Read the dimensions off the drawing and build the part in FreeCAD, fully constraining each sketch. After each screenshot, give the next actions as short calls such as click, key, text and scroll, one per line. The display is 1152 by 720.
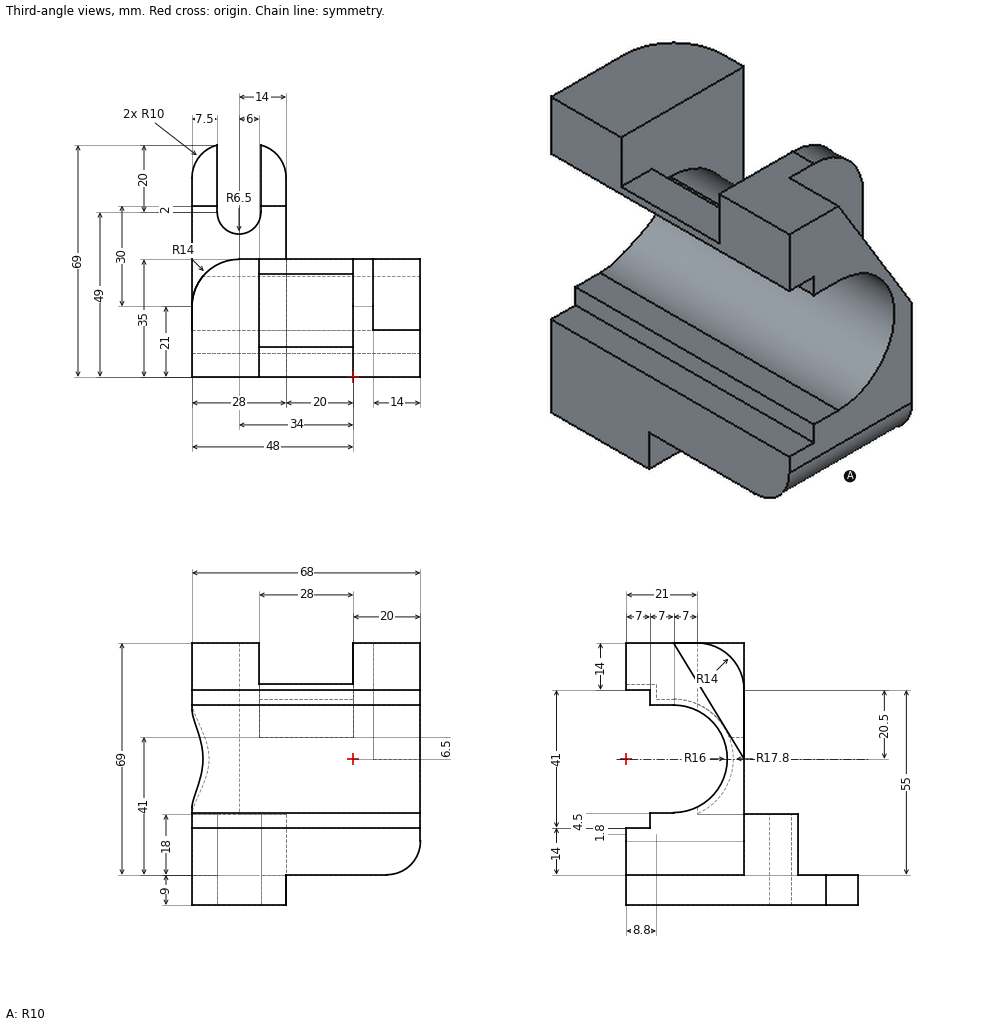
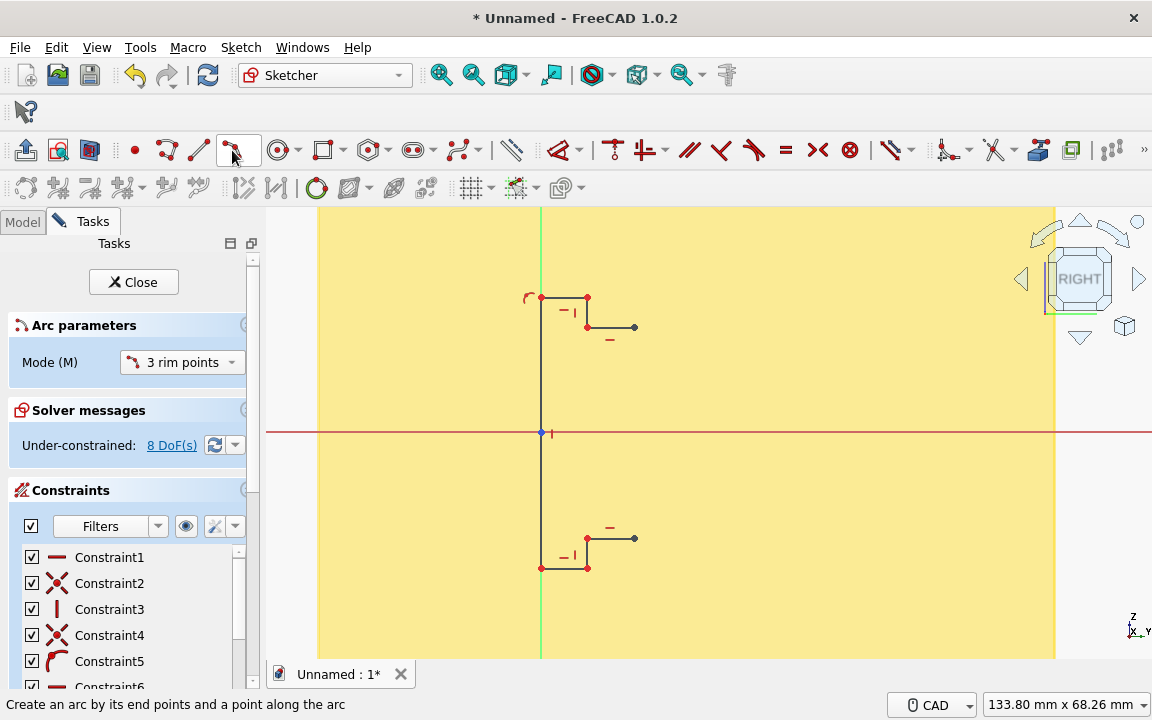
click(634, 539)
click(634, 328)
click(735, 465)
key(Escape)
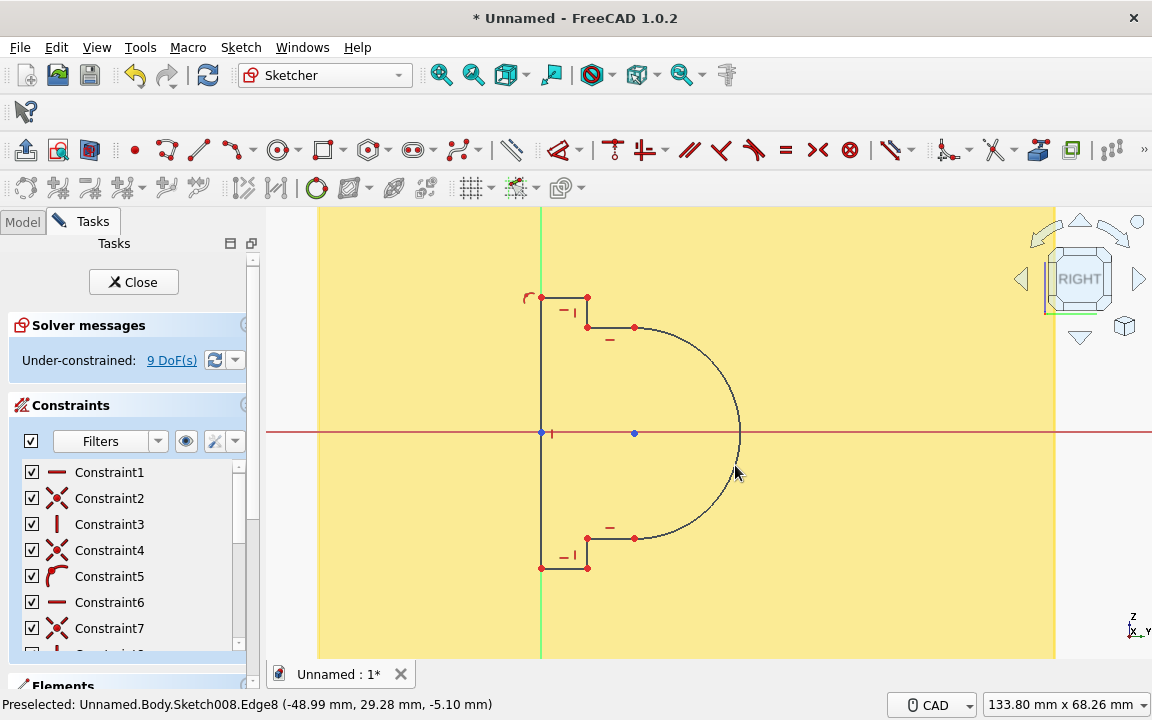
click(620, 328)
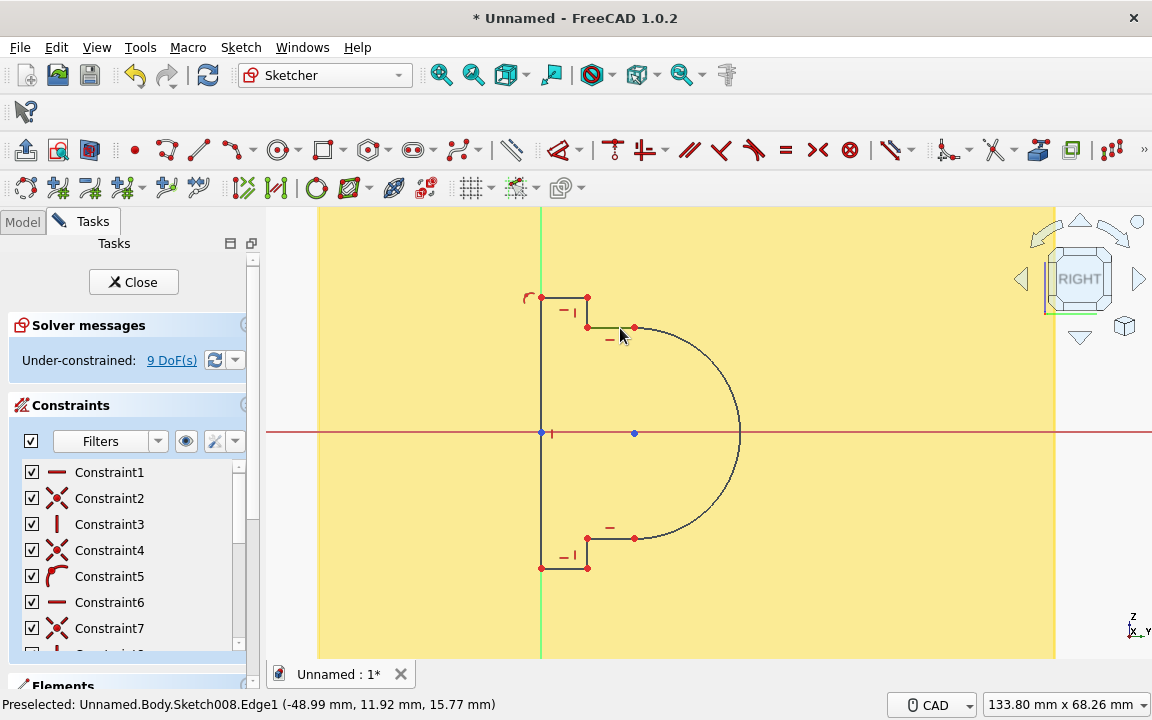
click(720, 496)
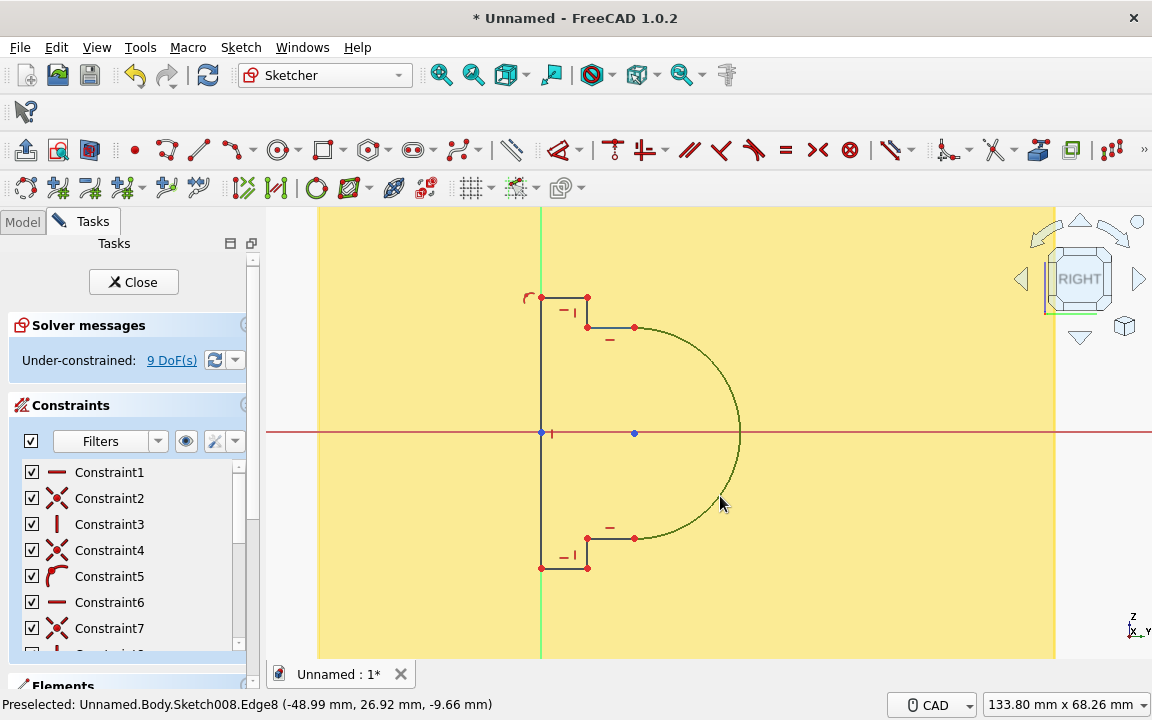
click(754, 150)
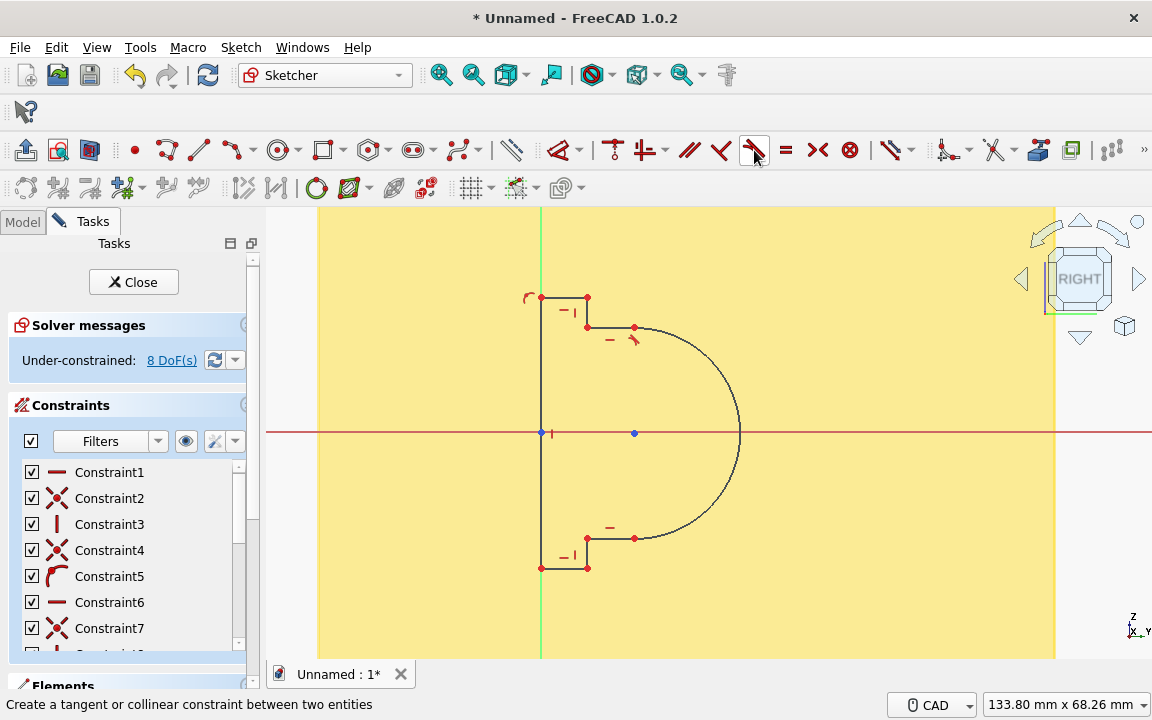
click(601, 539)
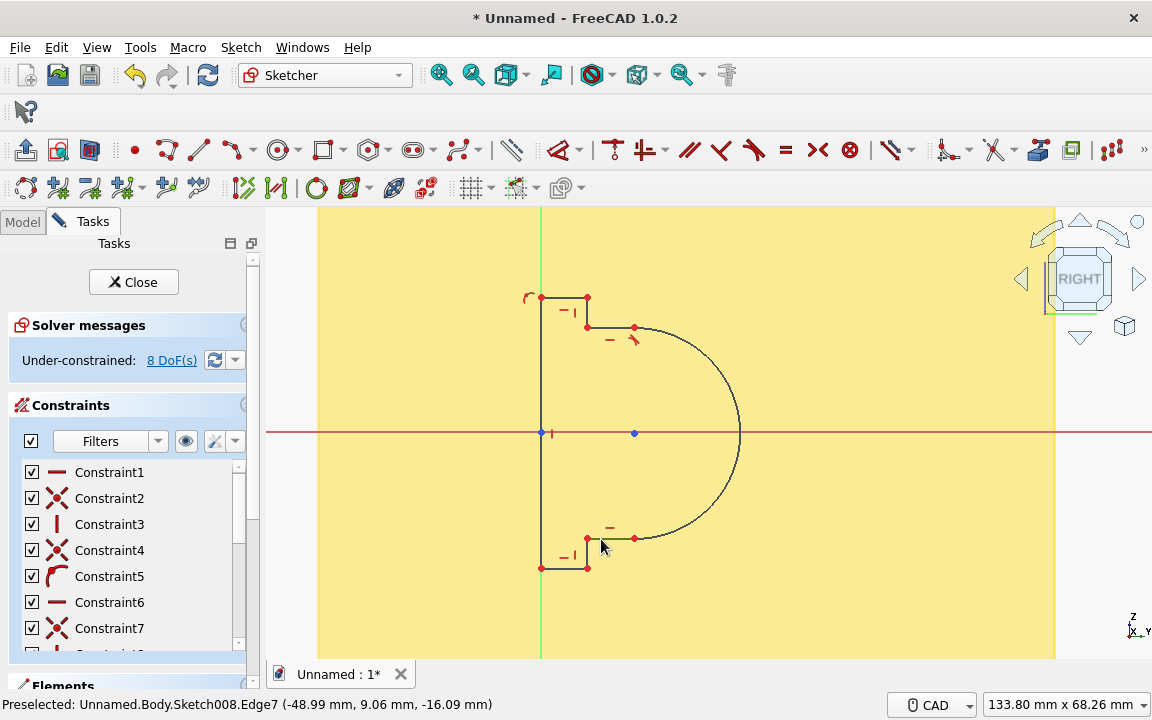
click(720, 496)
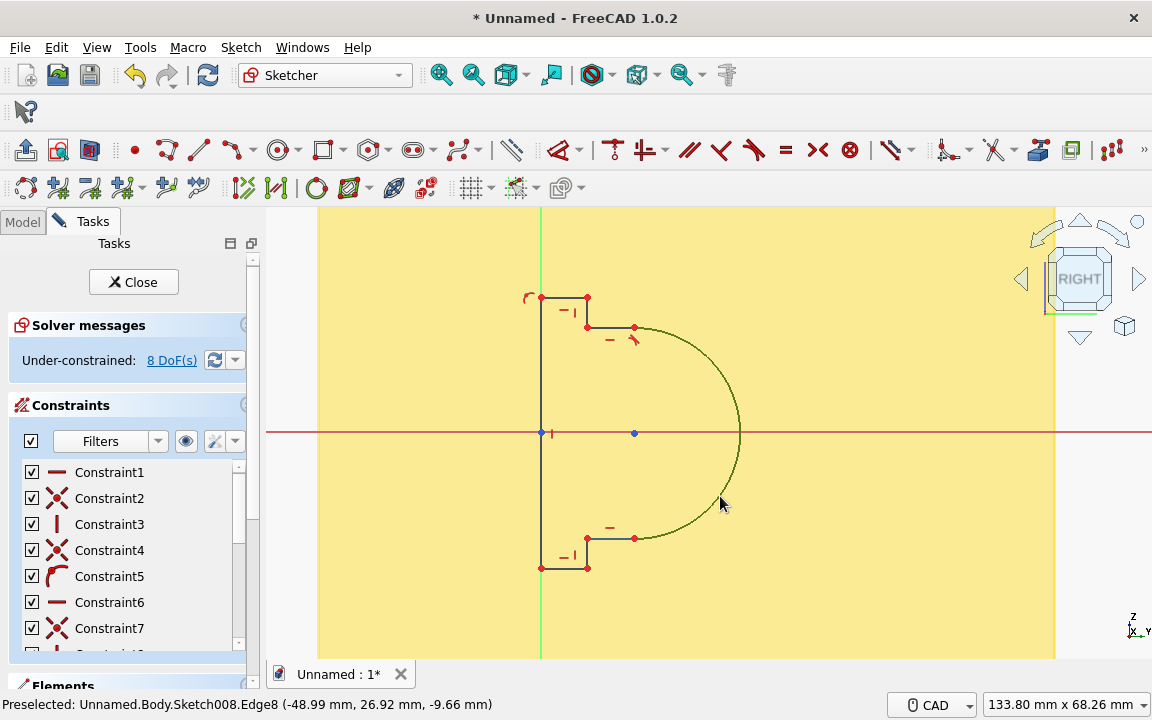
click(754, 150)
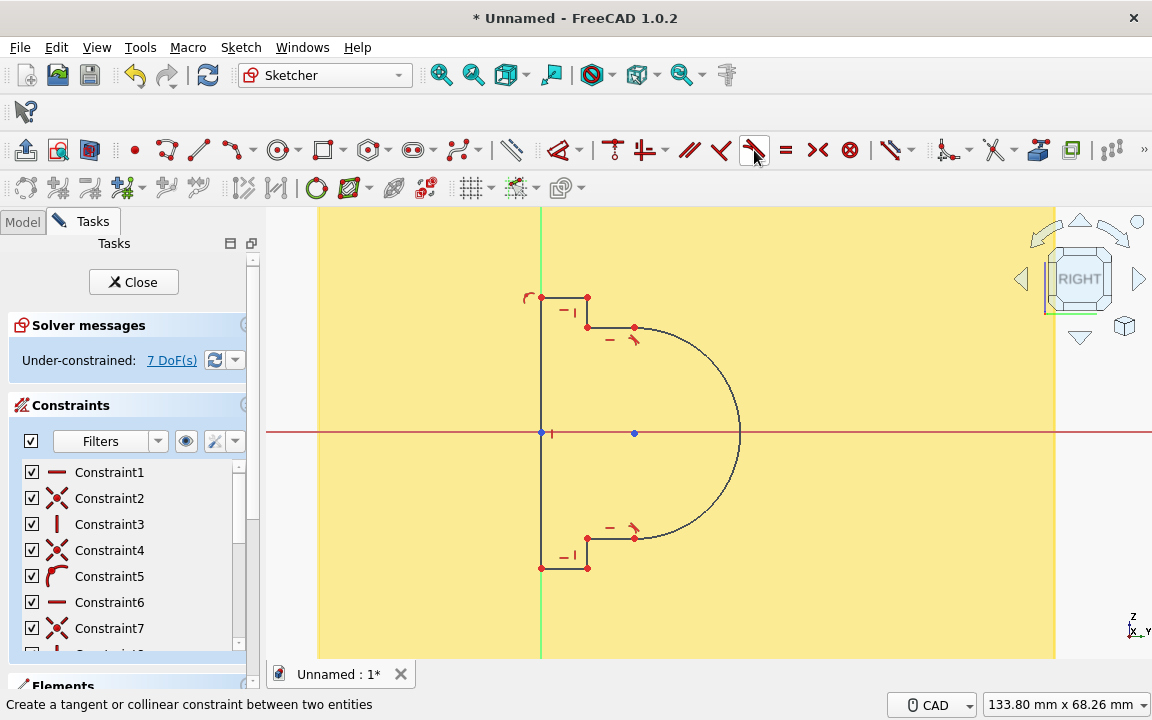
click(635, 434)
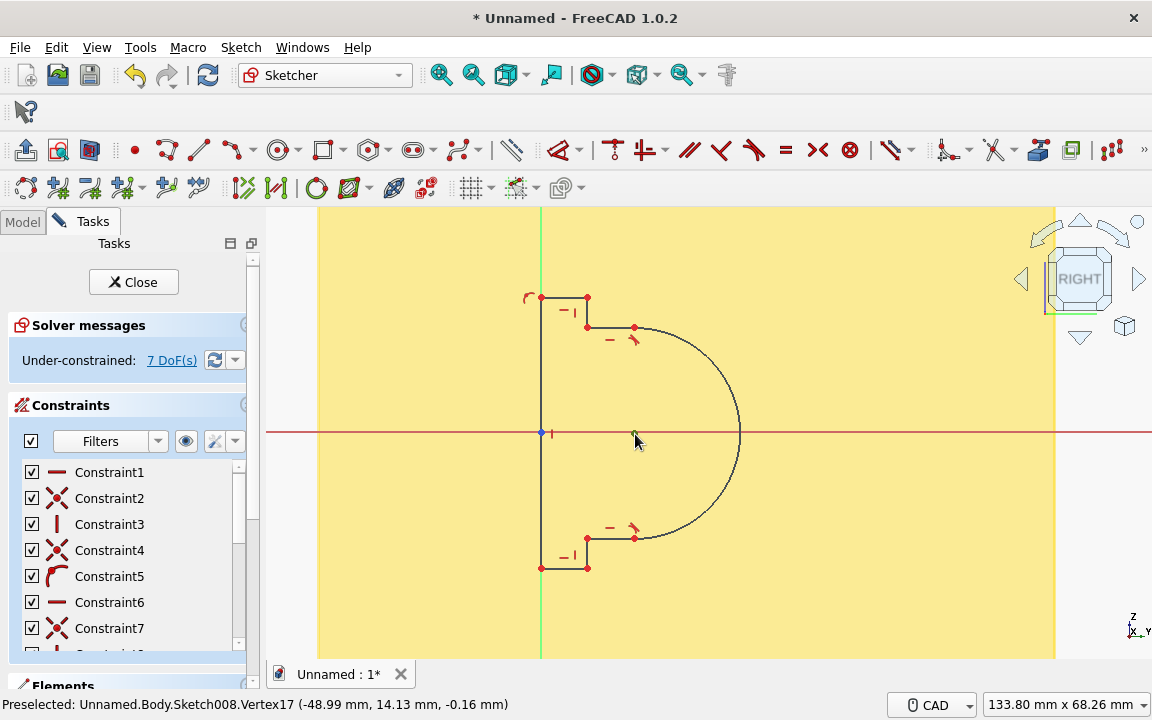
click(344, 432)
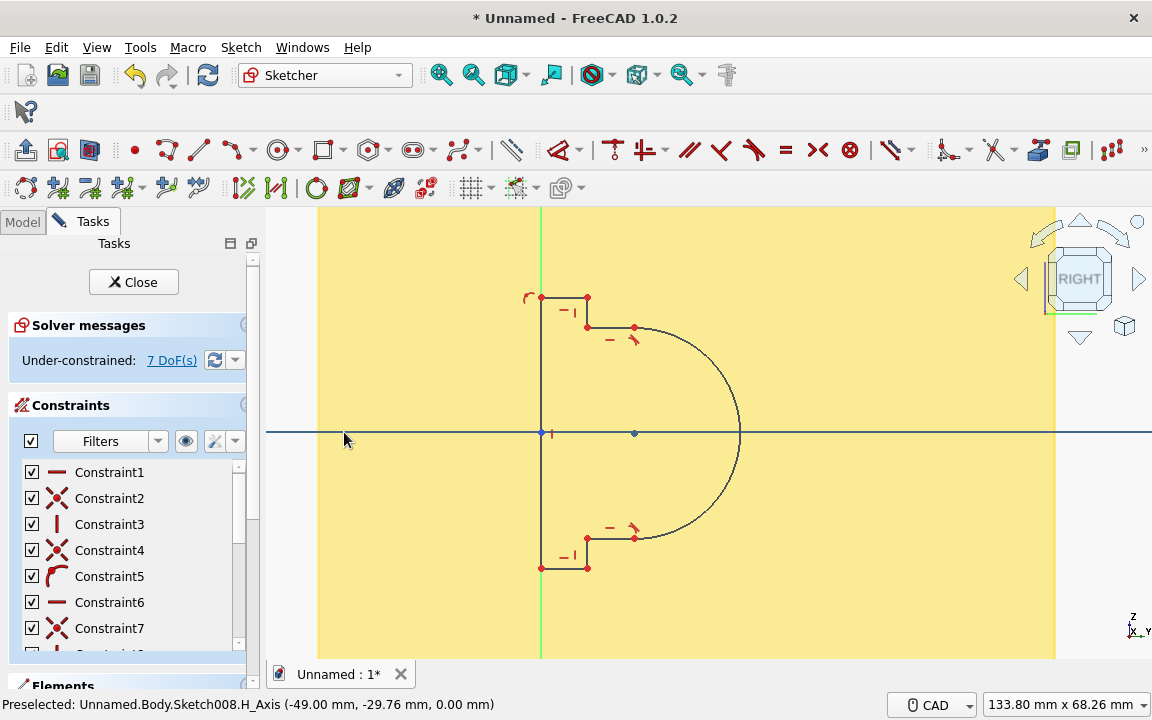
click(614, 150)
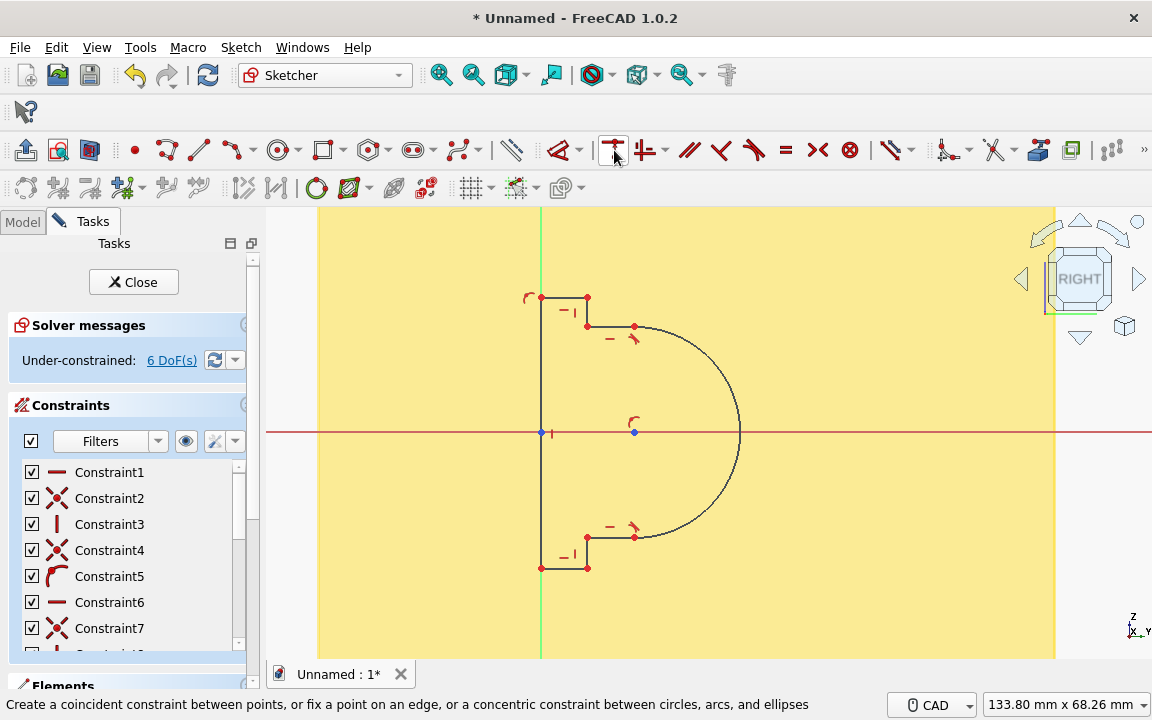
click(587, 298)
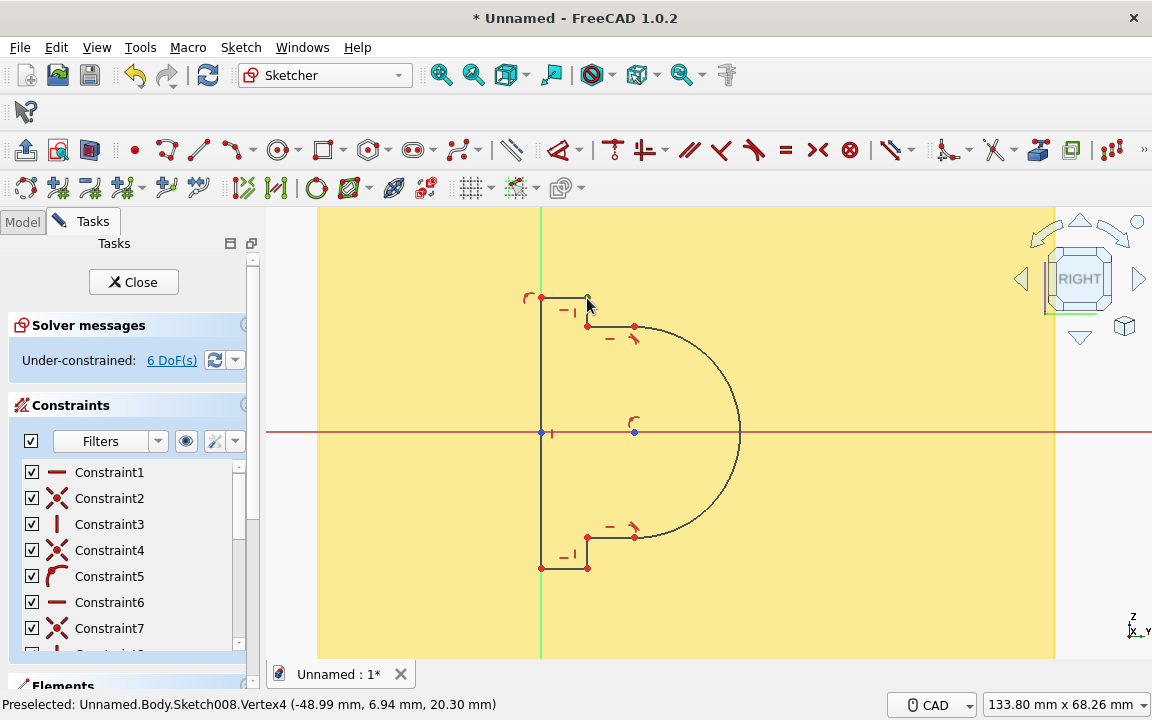
click(587, 569)